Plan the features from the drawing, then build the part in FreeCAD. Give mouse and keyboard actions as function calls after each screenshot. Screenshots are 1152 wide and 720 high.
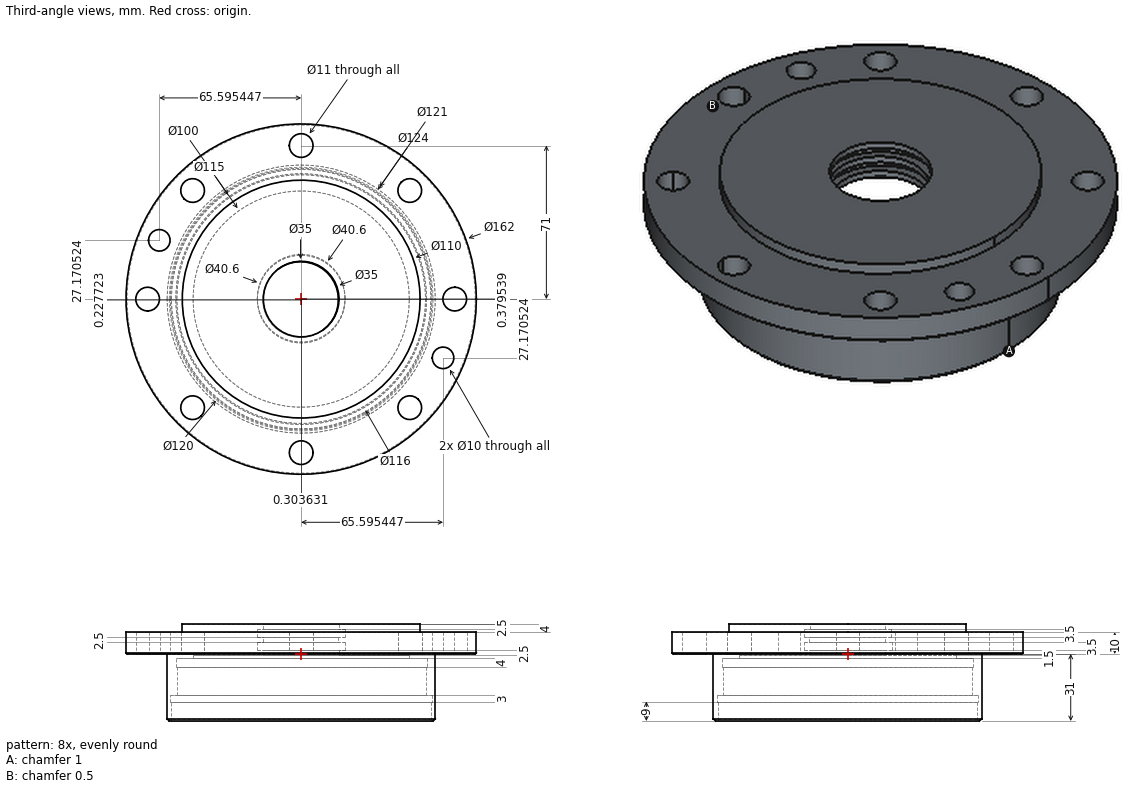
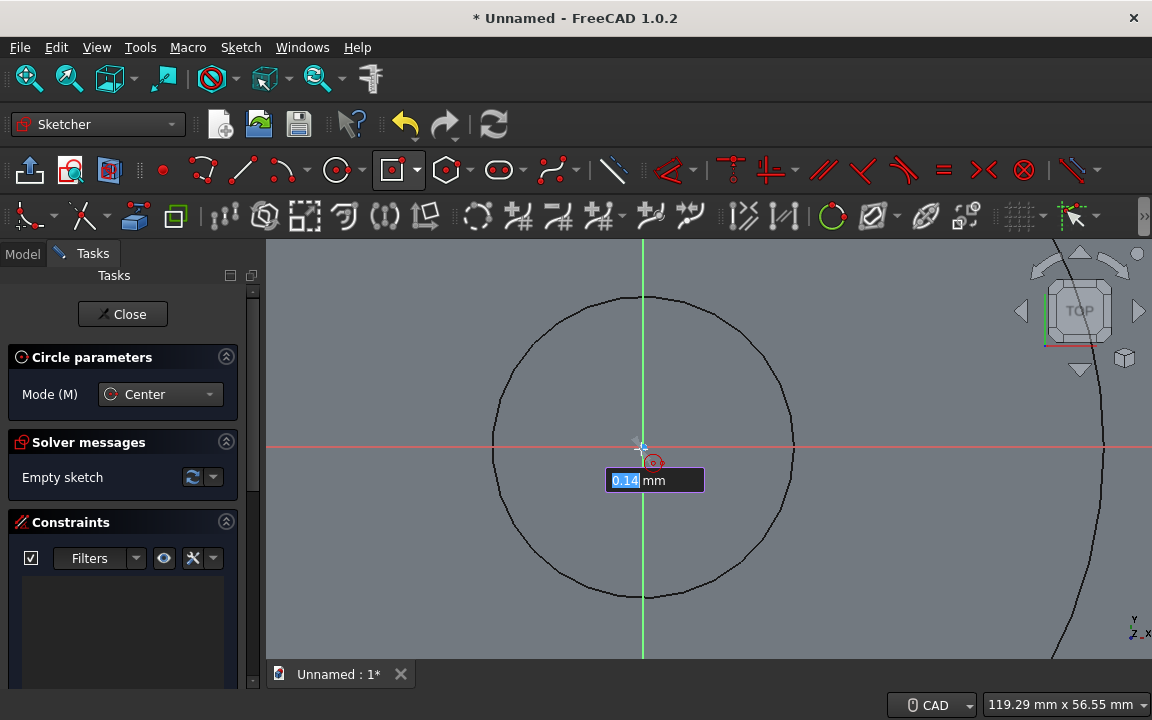
click(733, 357)
key(Escape)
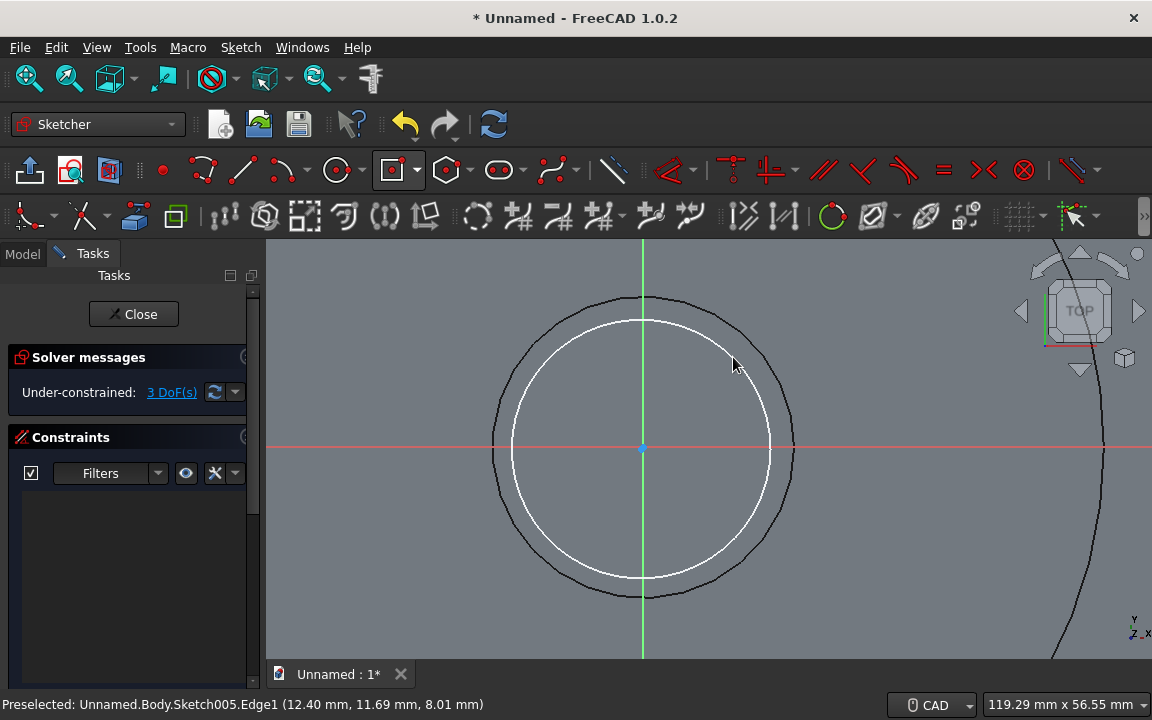
click(668, 170)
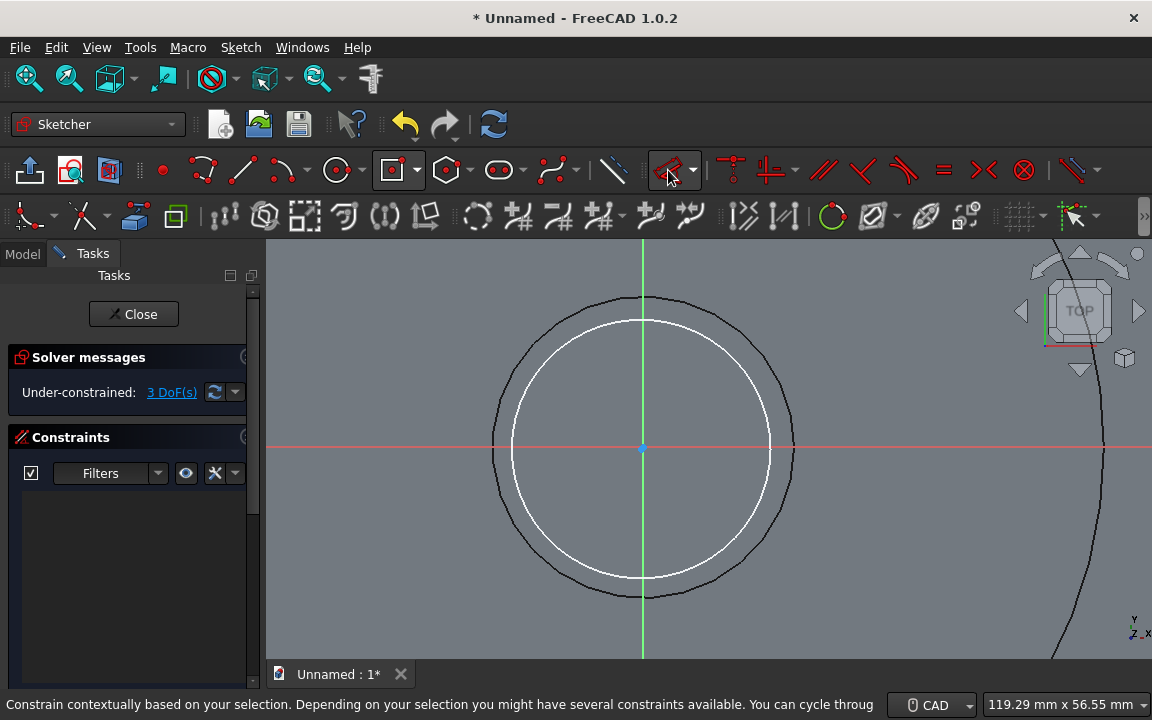
click(732, 357)
click(754, 334)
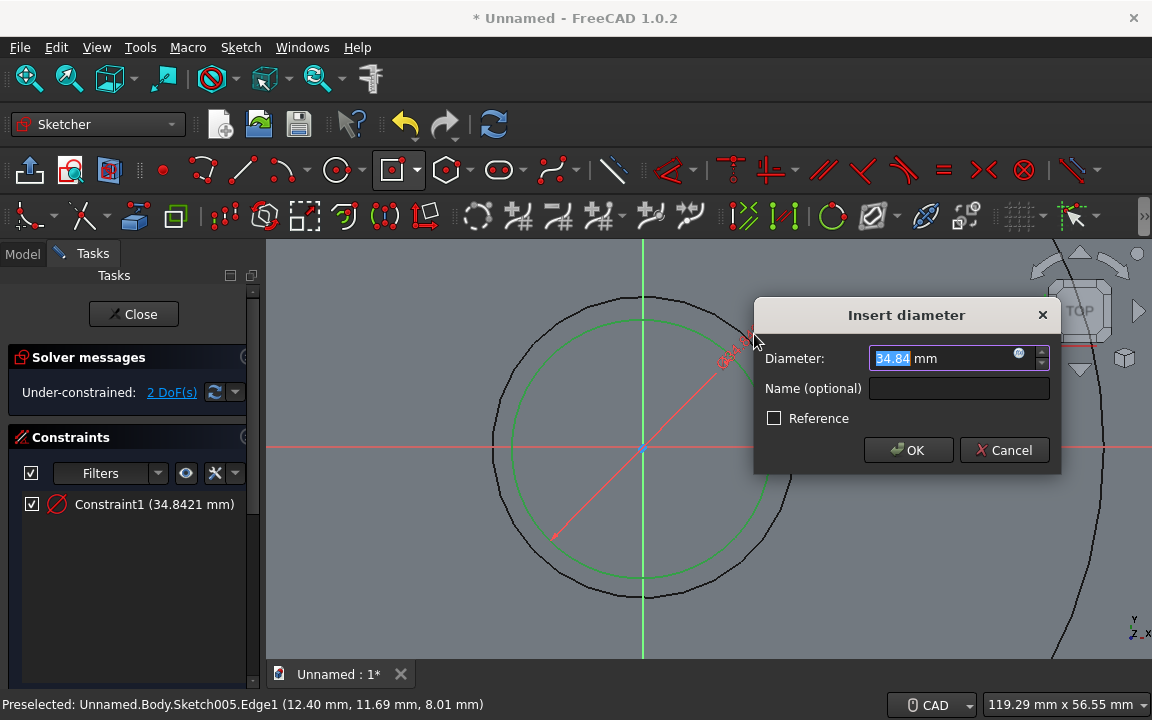
text(35)
key(Return)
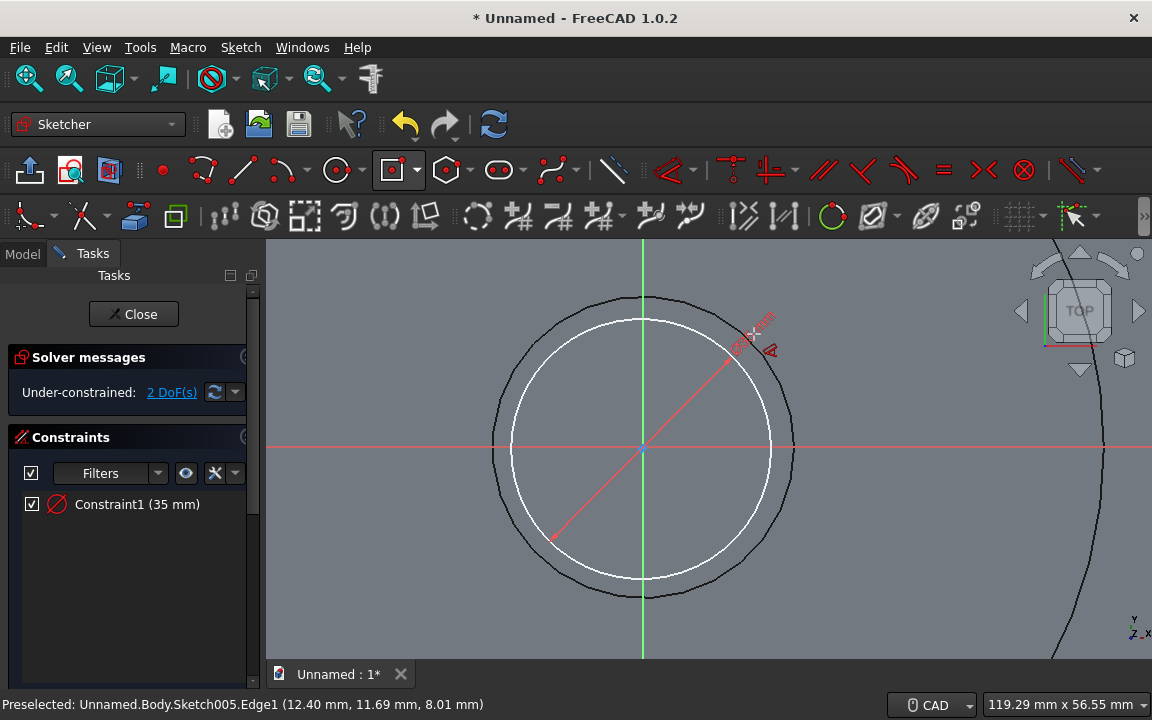
scroll(641, 449, up, 15)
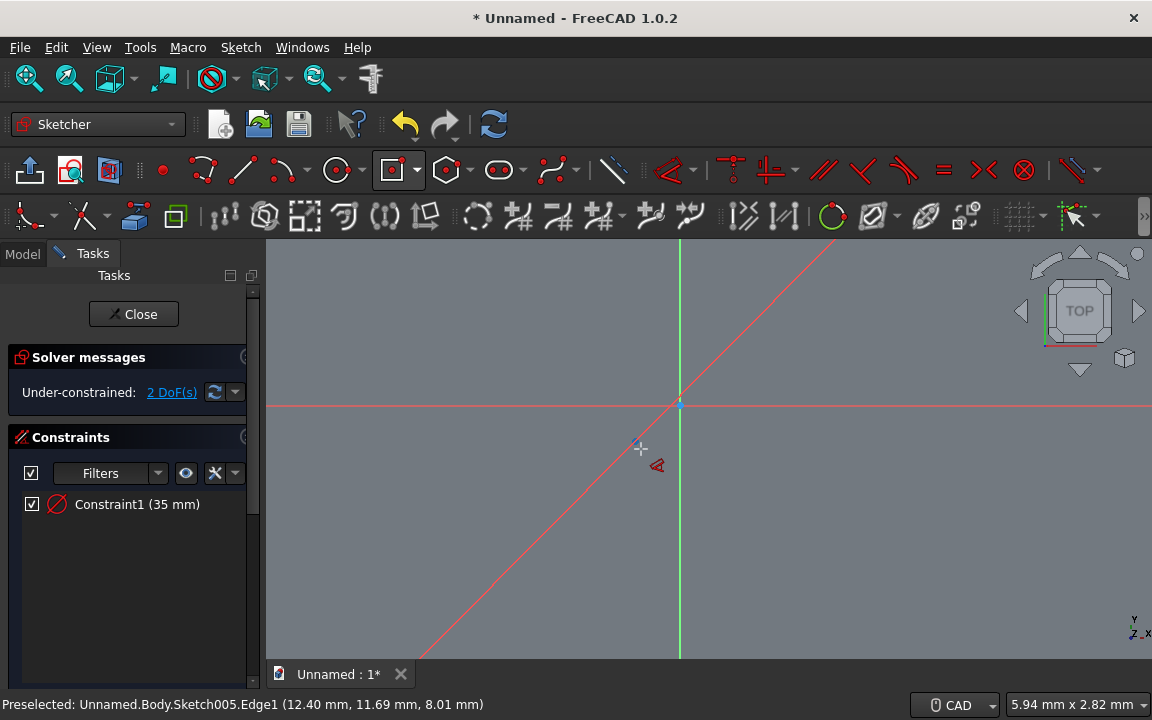
click(635, 441)
click(658, 372)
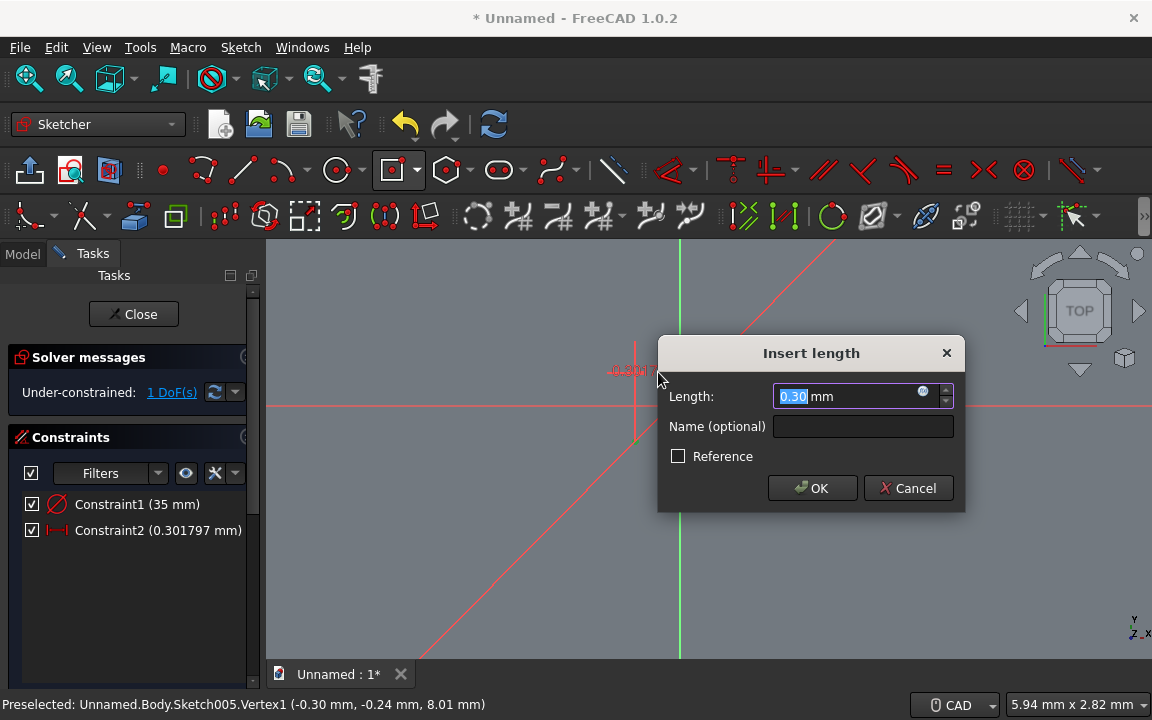
text(0.303631)
key(Return)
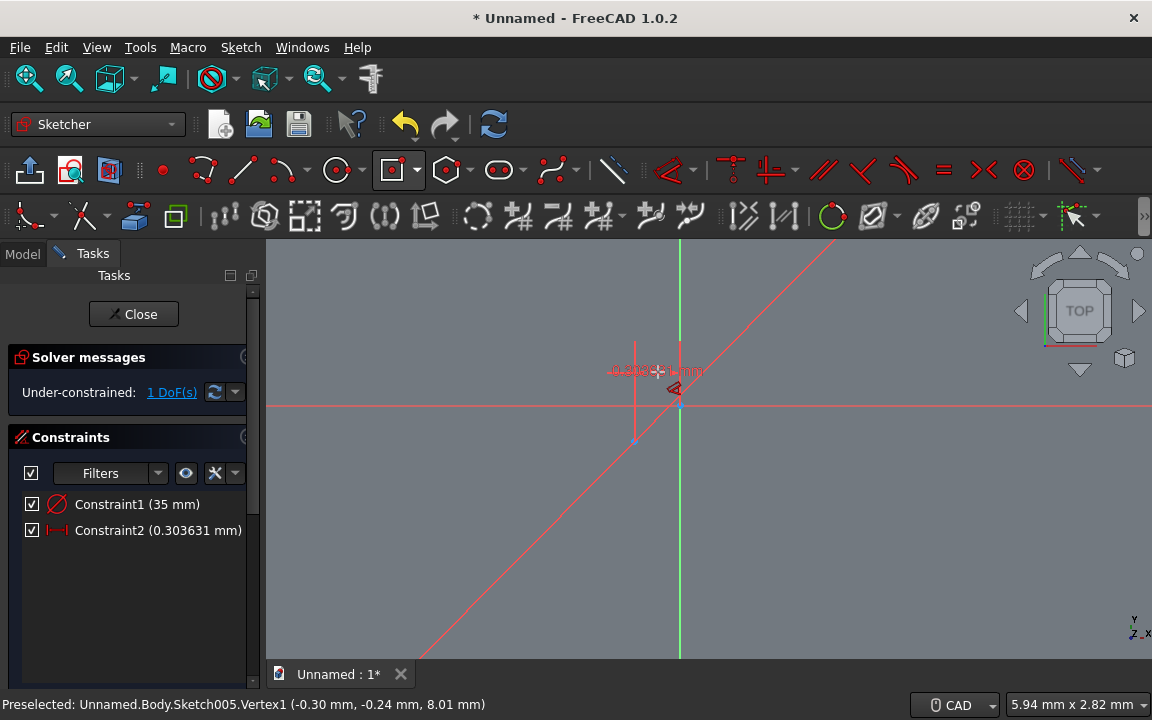
click(635, 441)
click(714, 424)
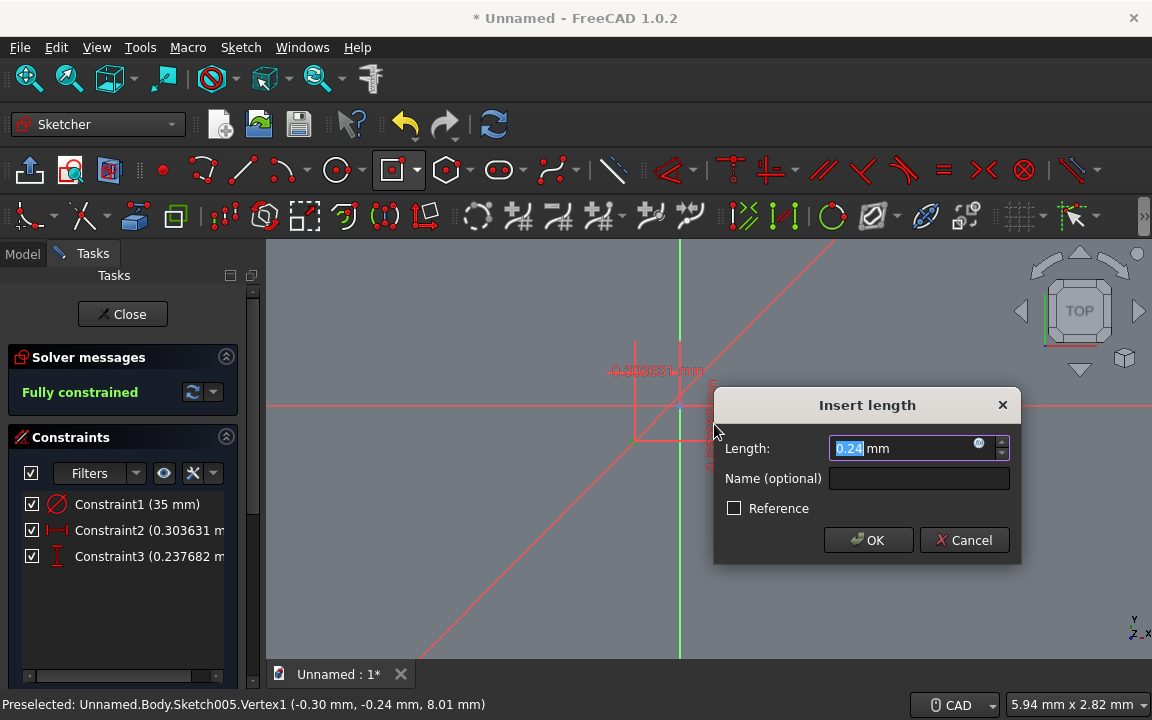
text(0.227723)
key(Return)
key(Escape)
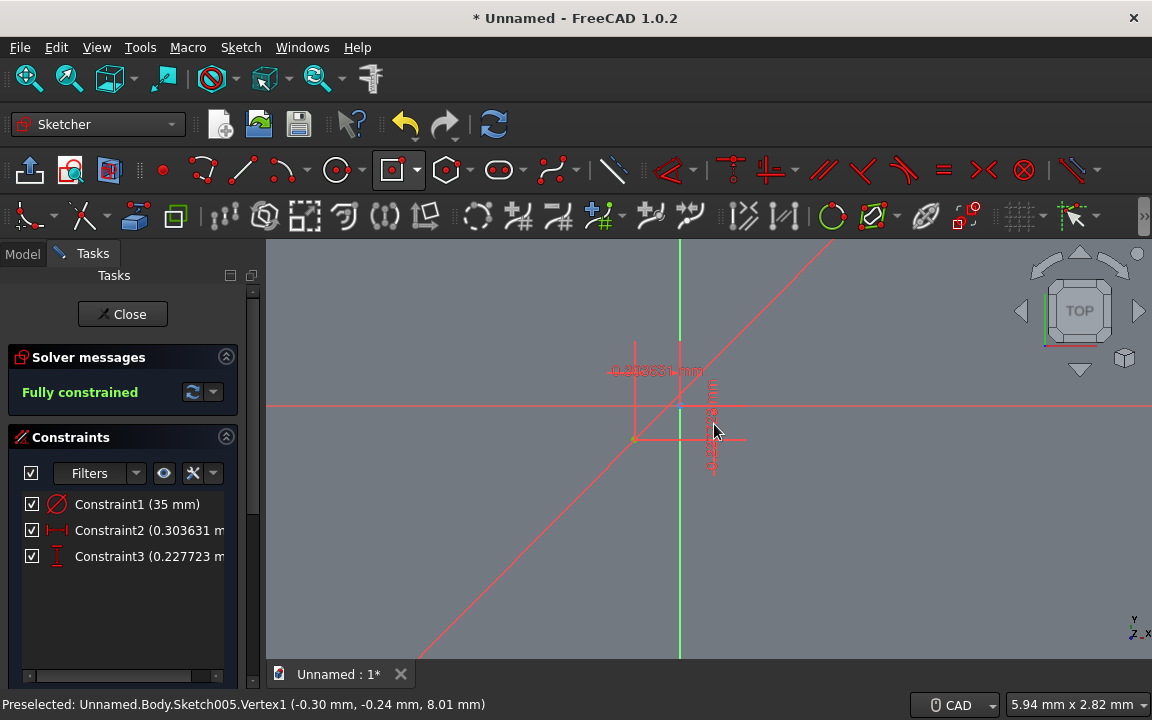
click(123, 314)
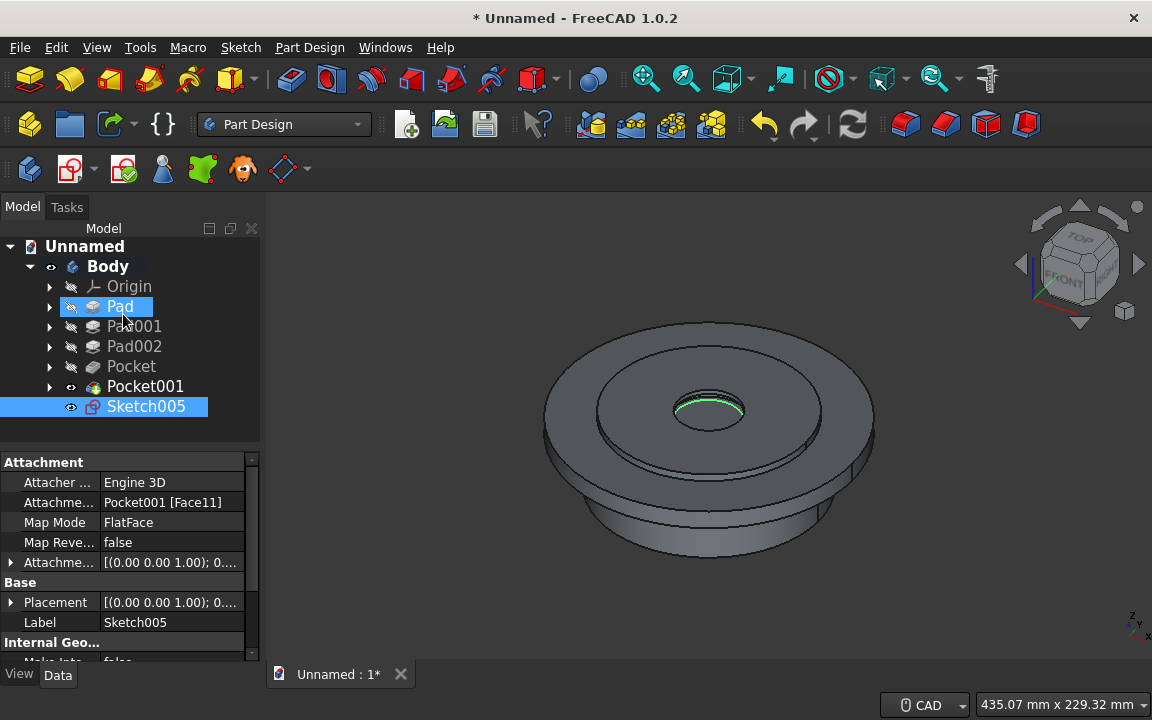
click(292, 80)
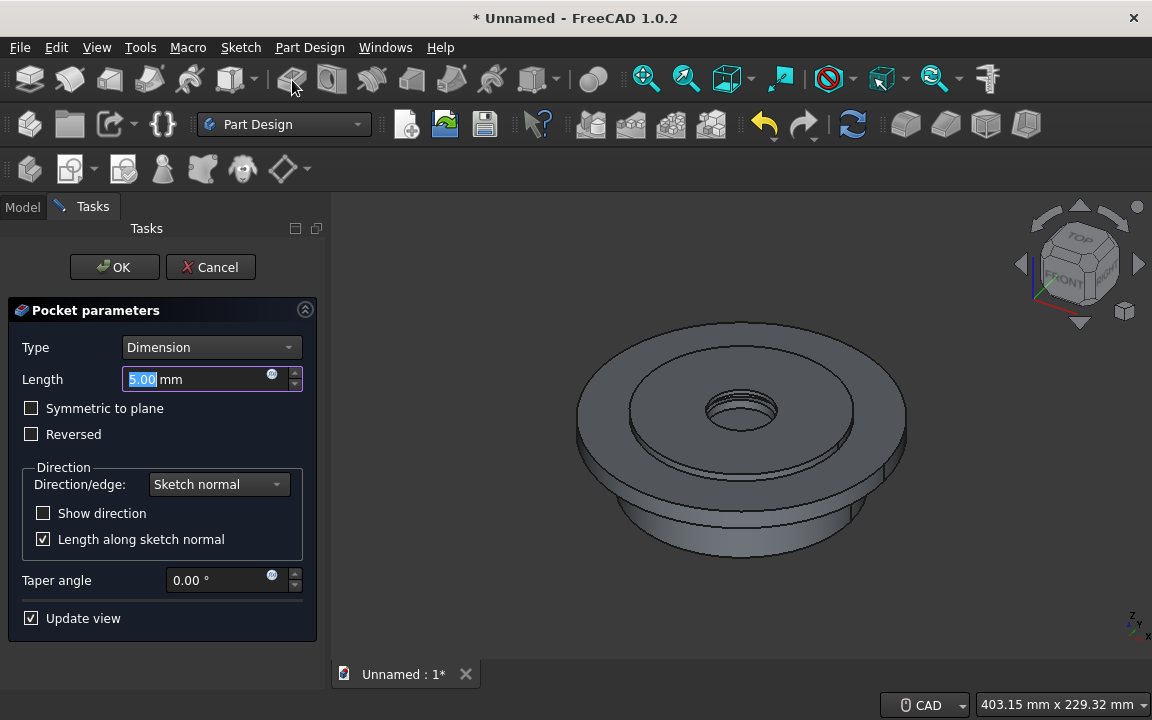
text(2.5)
key(Tab)